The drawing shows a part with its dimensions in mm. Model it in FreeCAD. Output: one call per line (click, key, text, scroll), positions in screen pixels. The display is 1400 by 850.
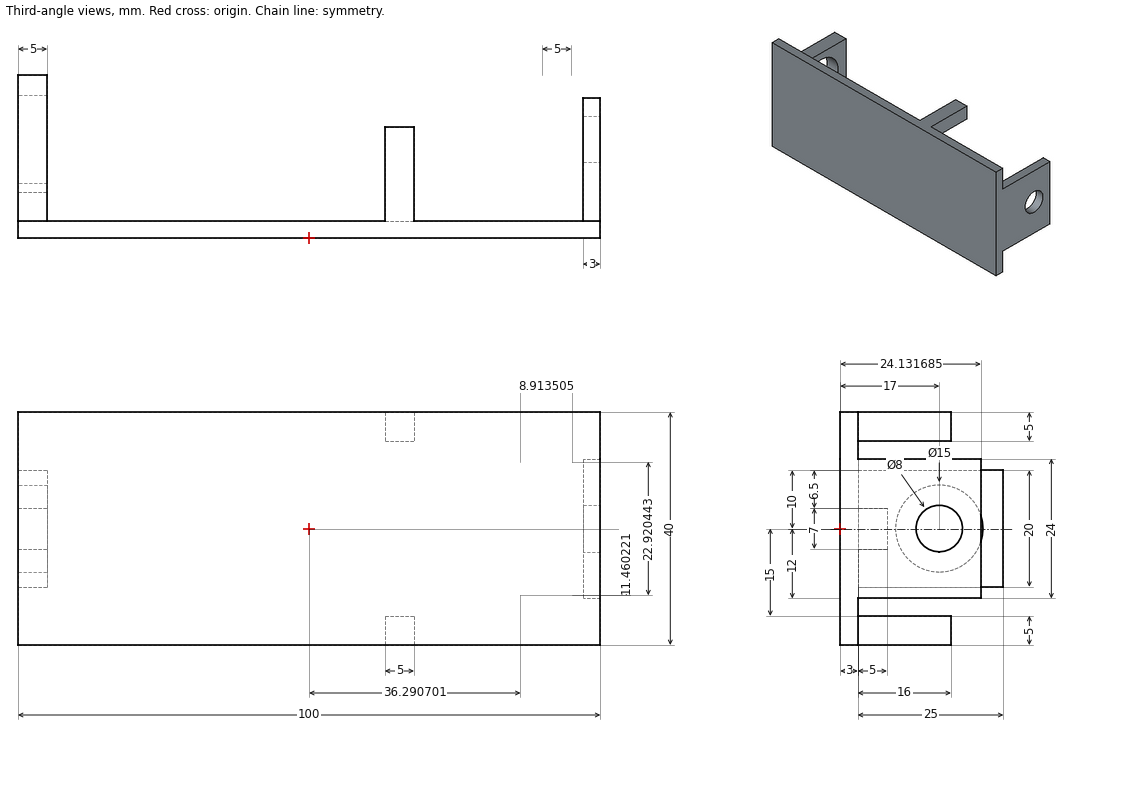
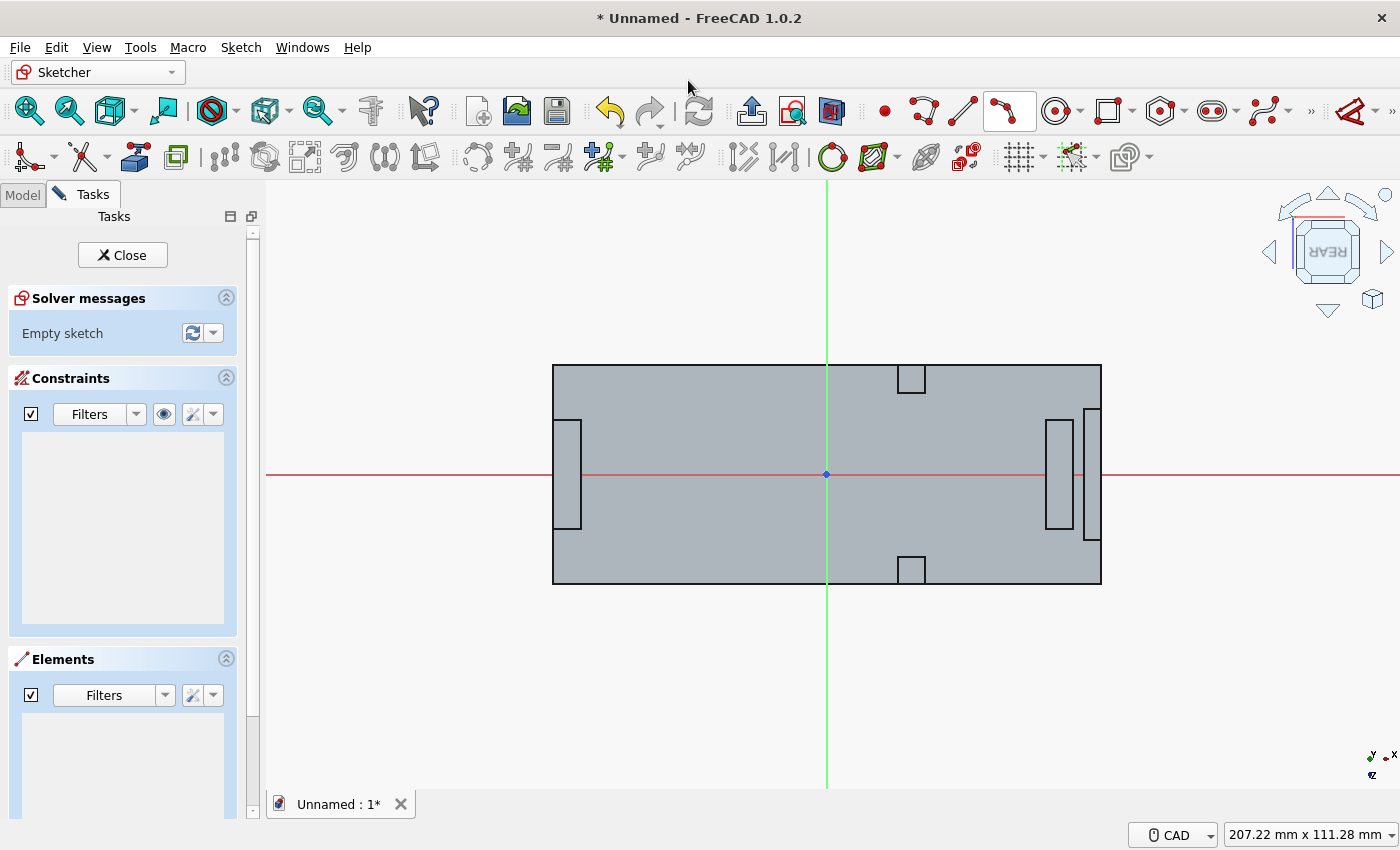
scroll(1059, 469, up, 5)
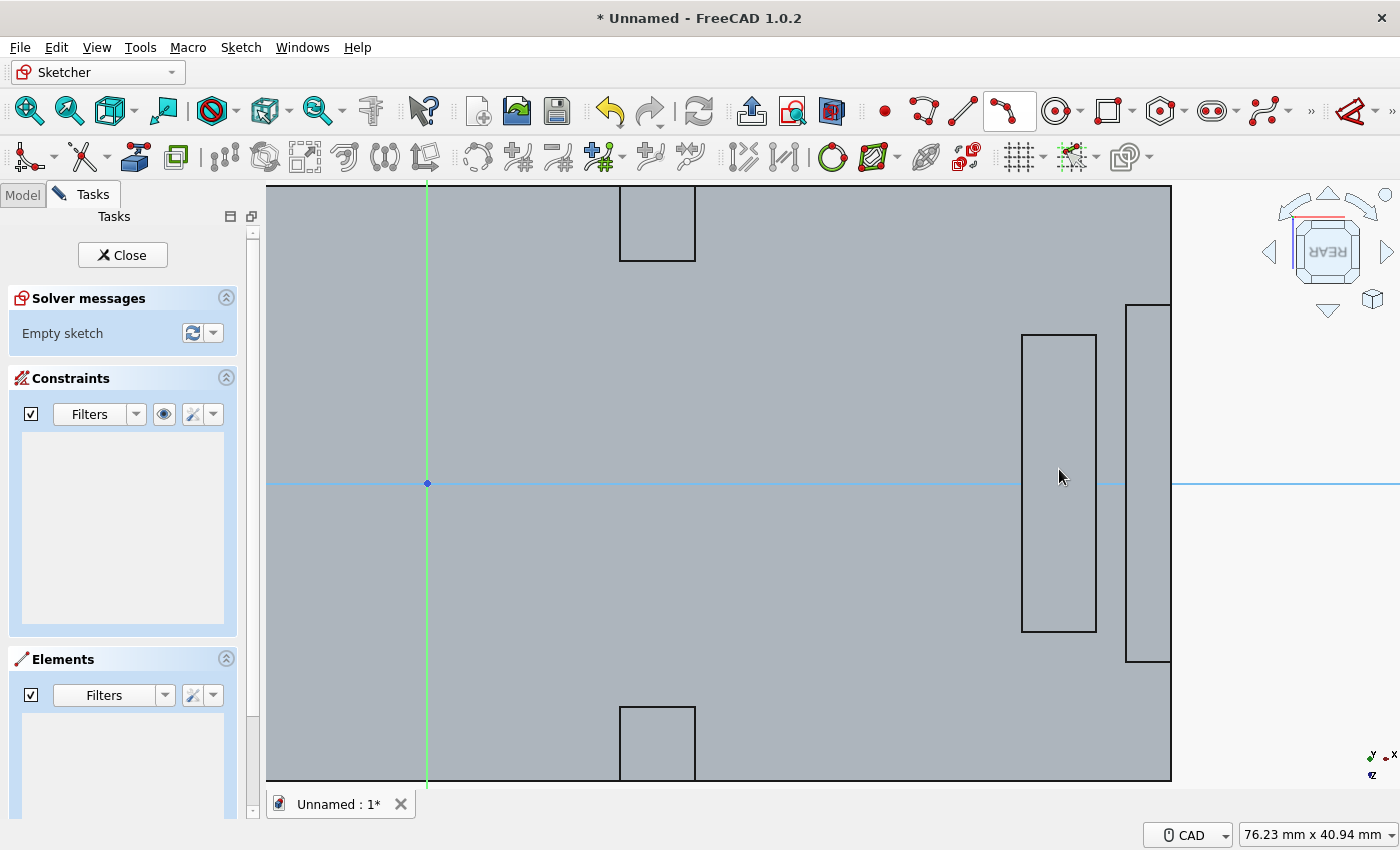
click(1108, 112)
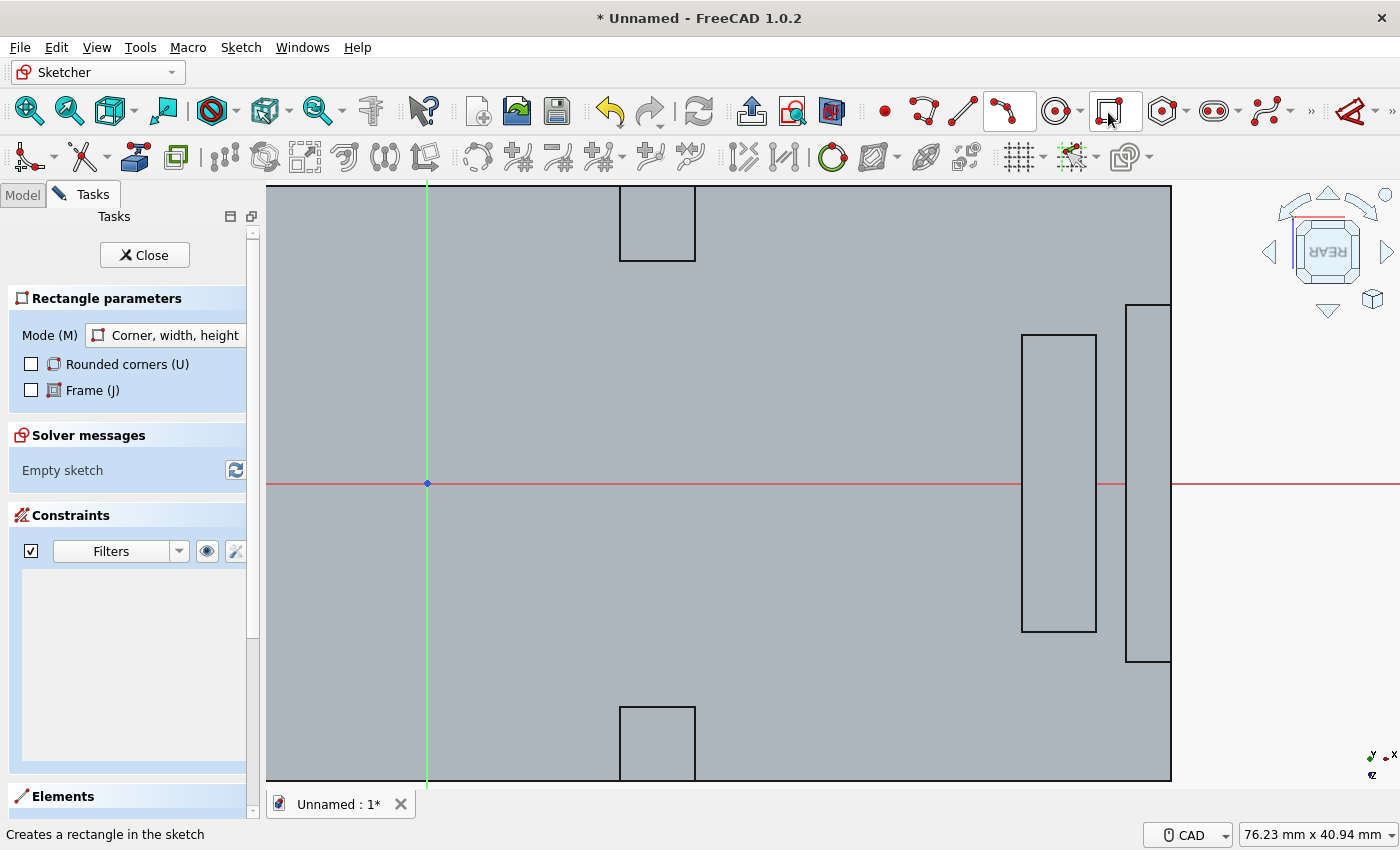
click(967, 313)
move(1099, 654)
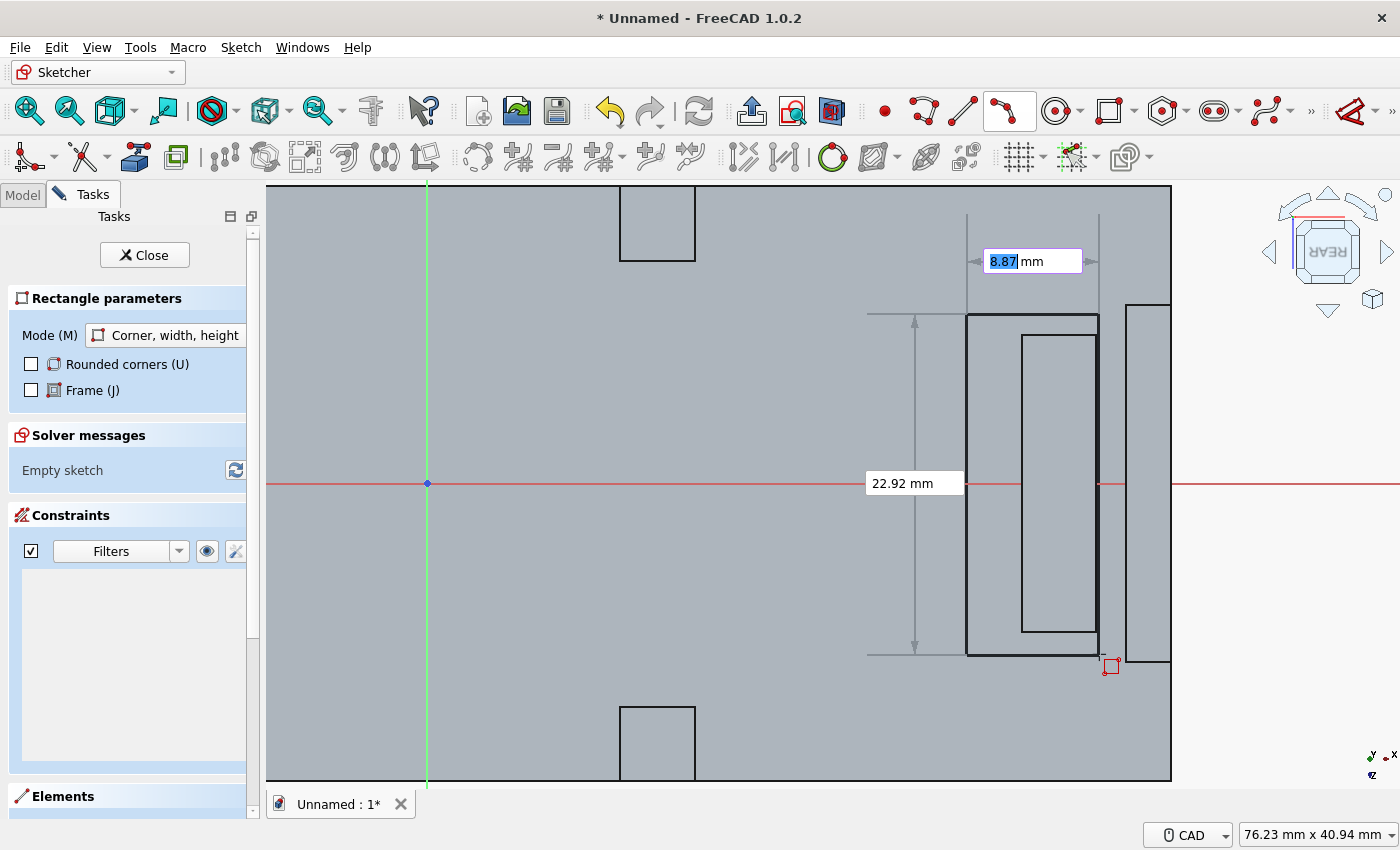
text(8.913505)
key(Tab)
text(22.920443)
key(Return)
key(Escape)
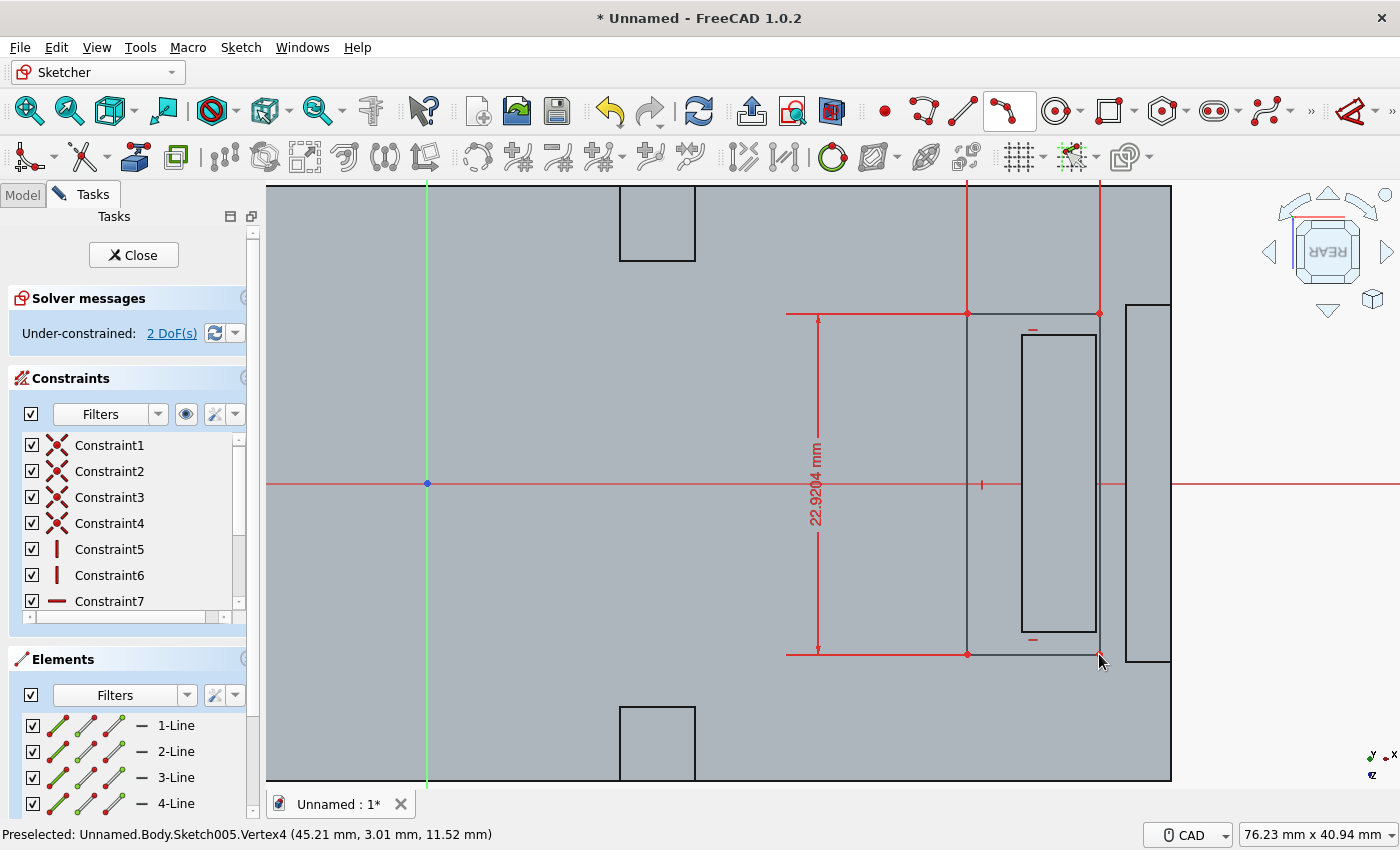
click(1350, 112)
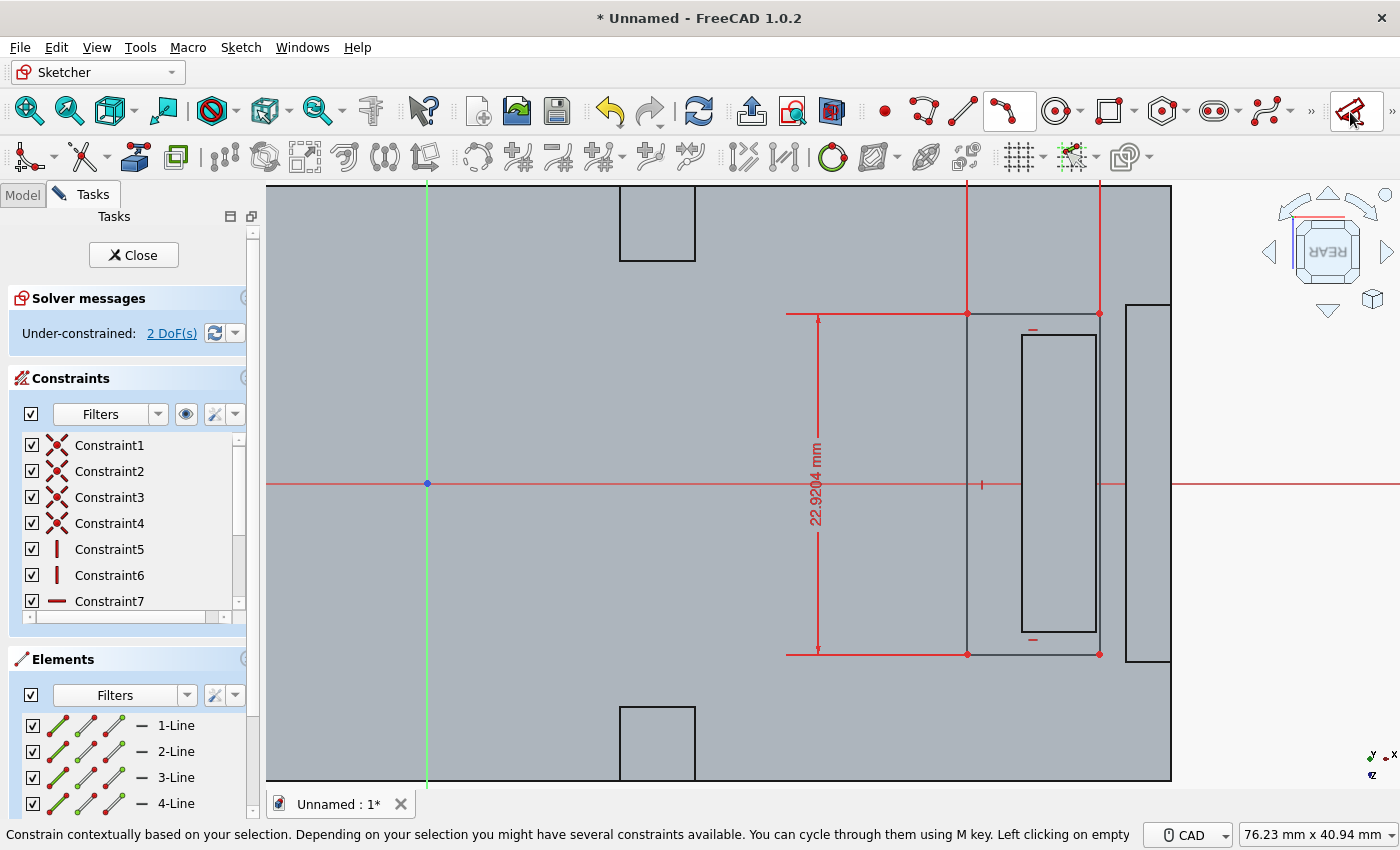
click(967, 314)
click(697, 280)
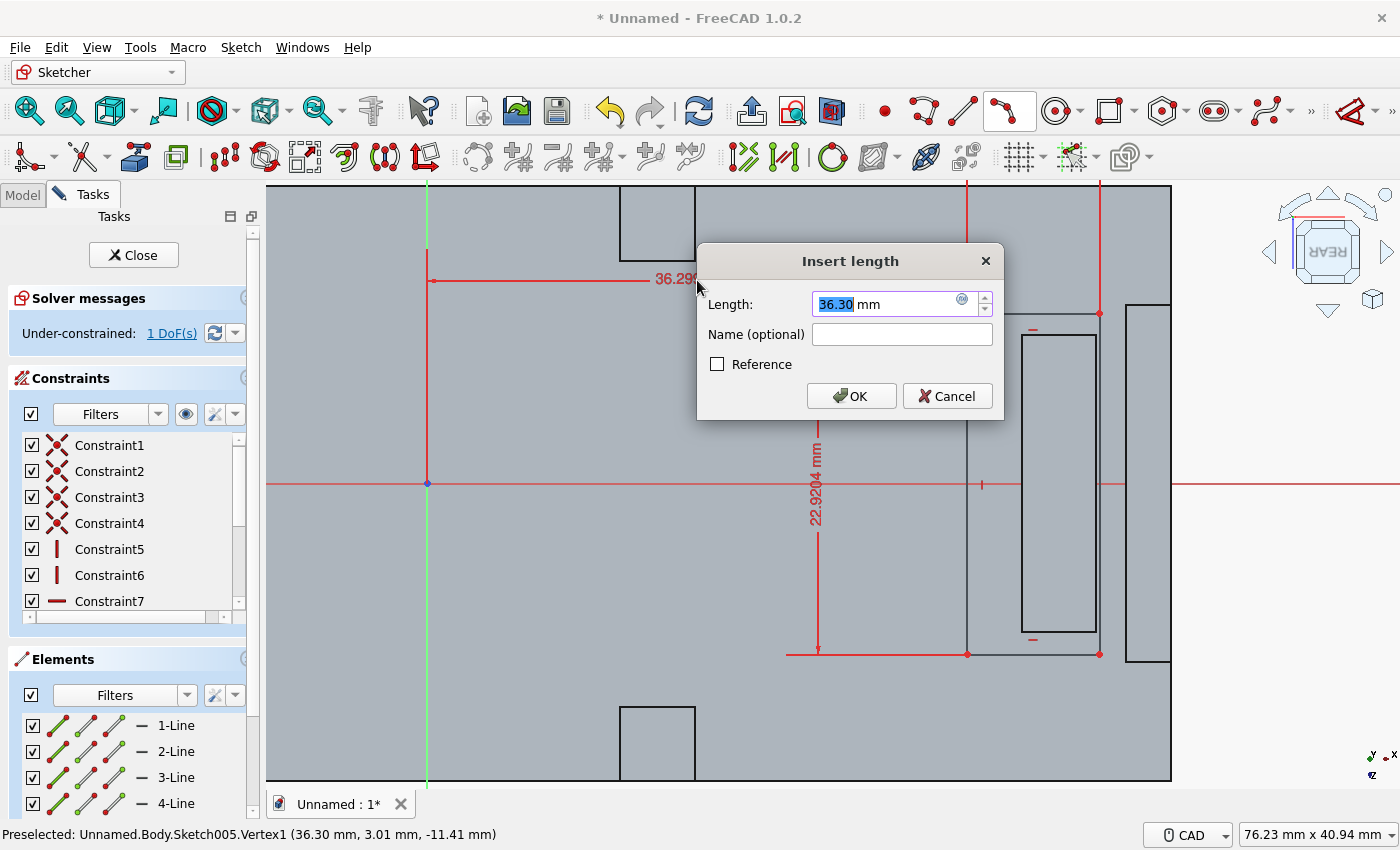
text(36.290701)
key(Return)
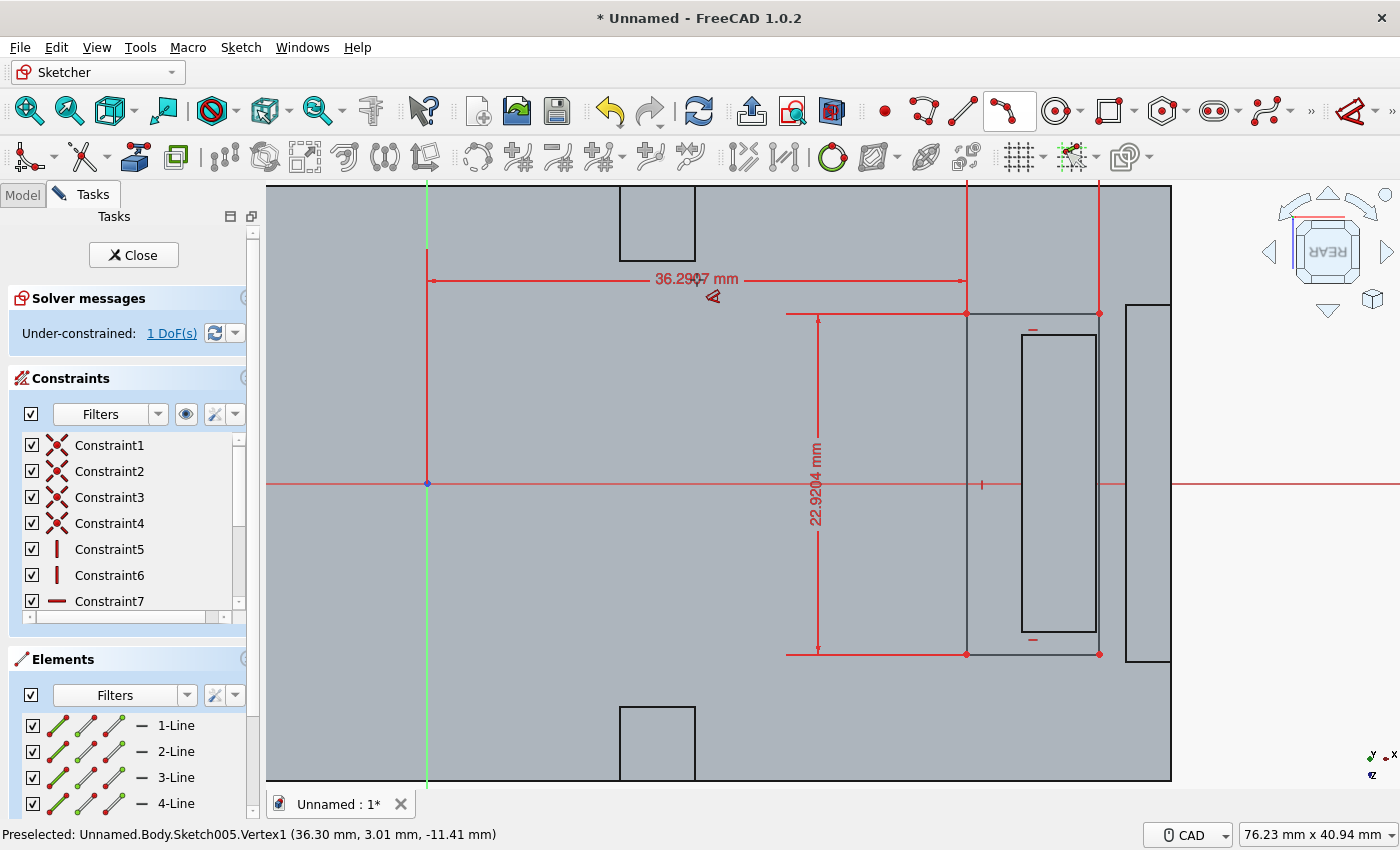
click(967, 314)
click(393, 399)